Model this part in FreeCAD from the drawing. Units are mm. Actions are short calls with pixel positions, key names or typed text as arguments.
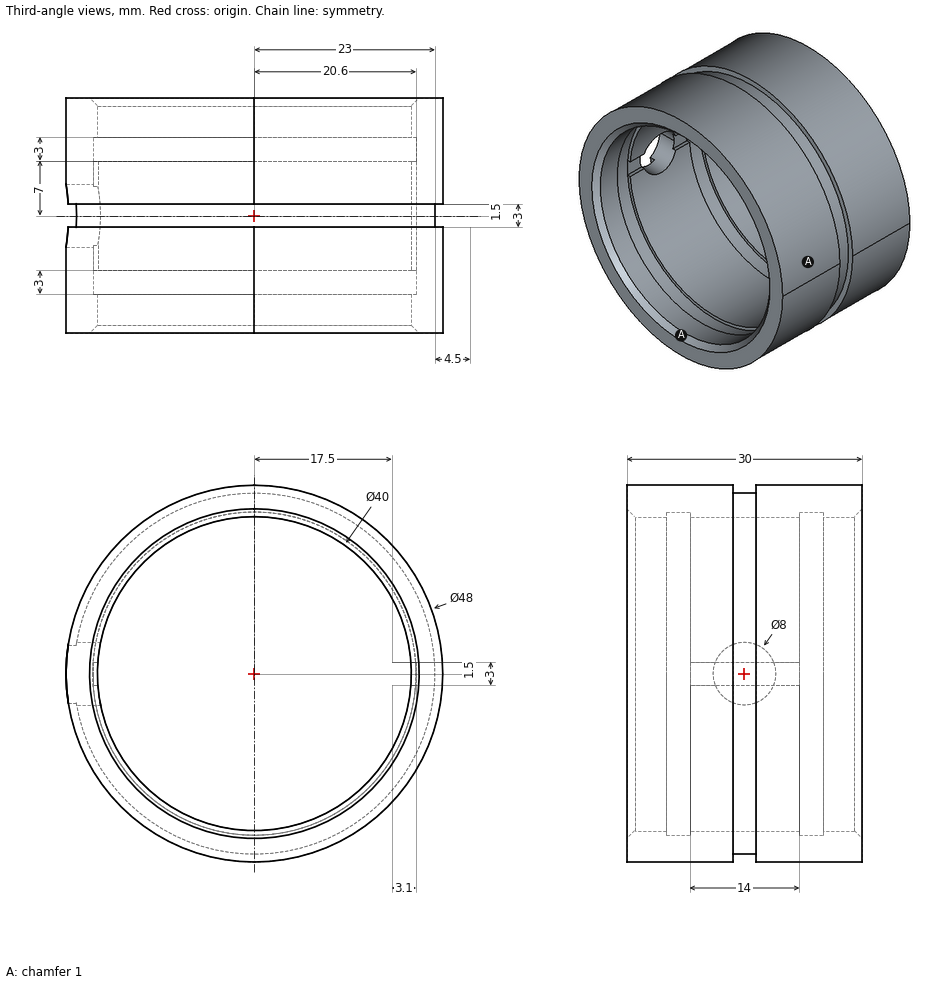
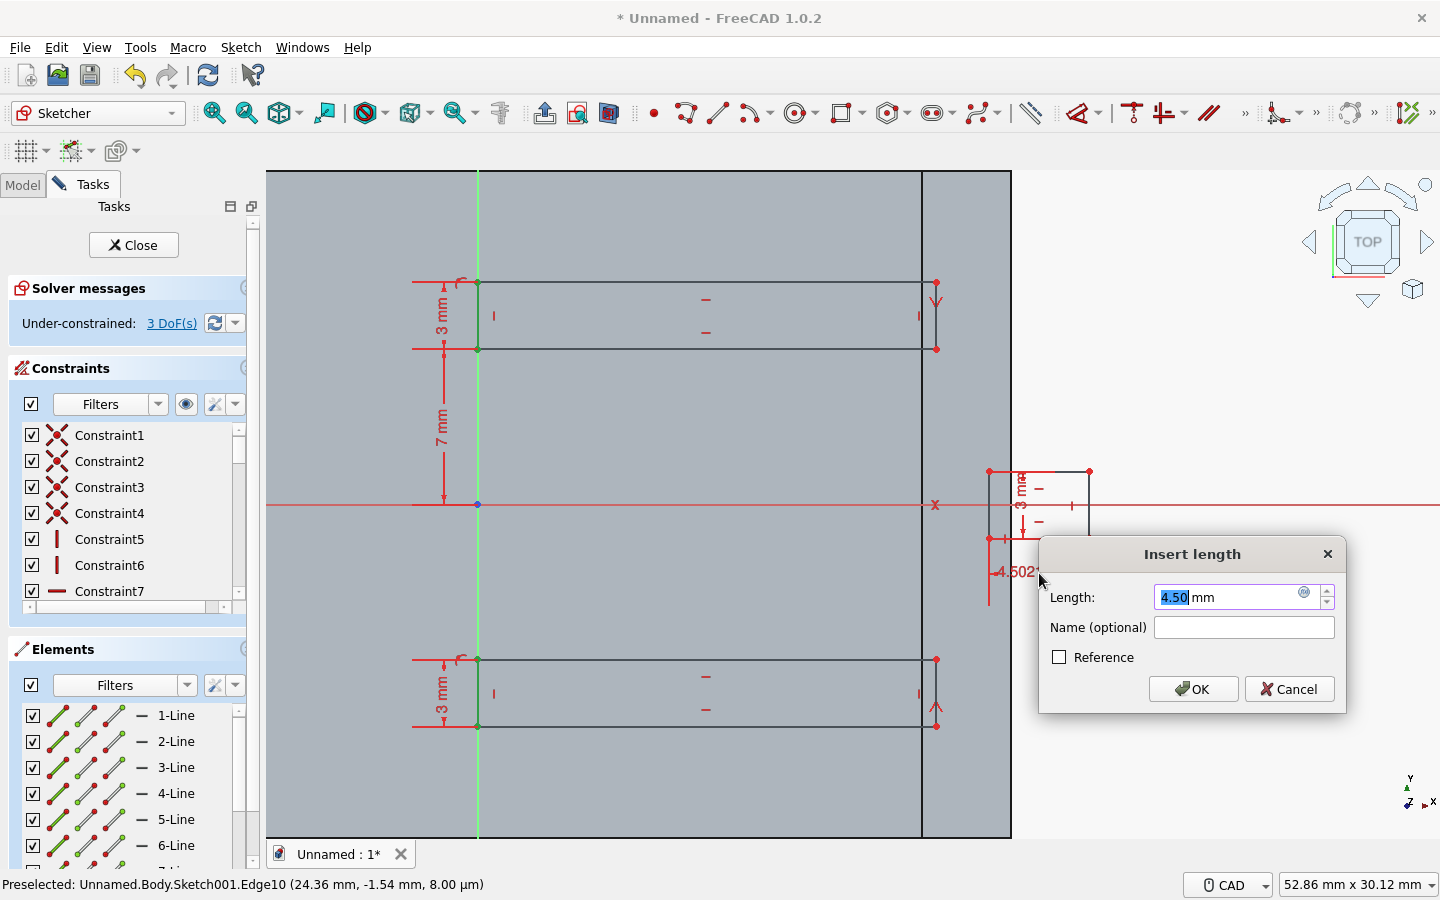
text(4.5)
key(Return)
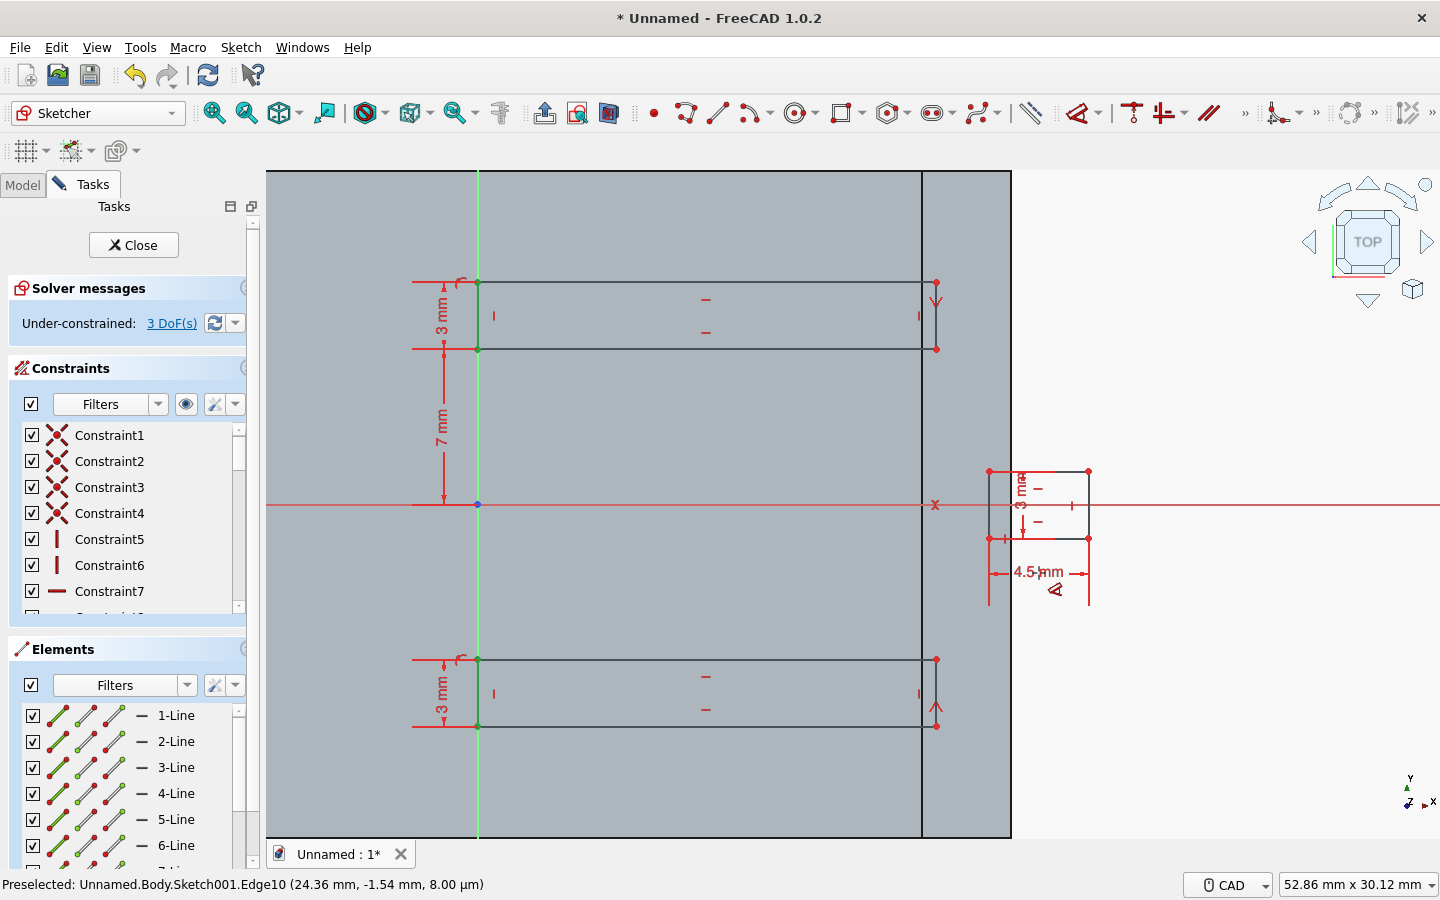
click(989, 472)
click(733, 438)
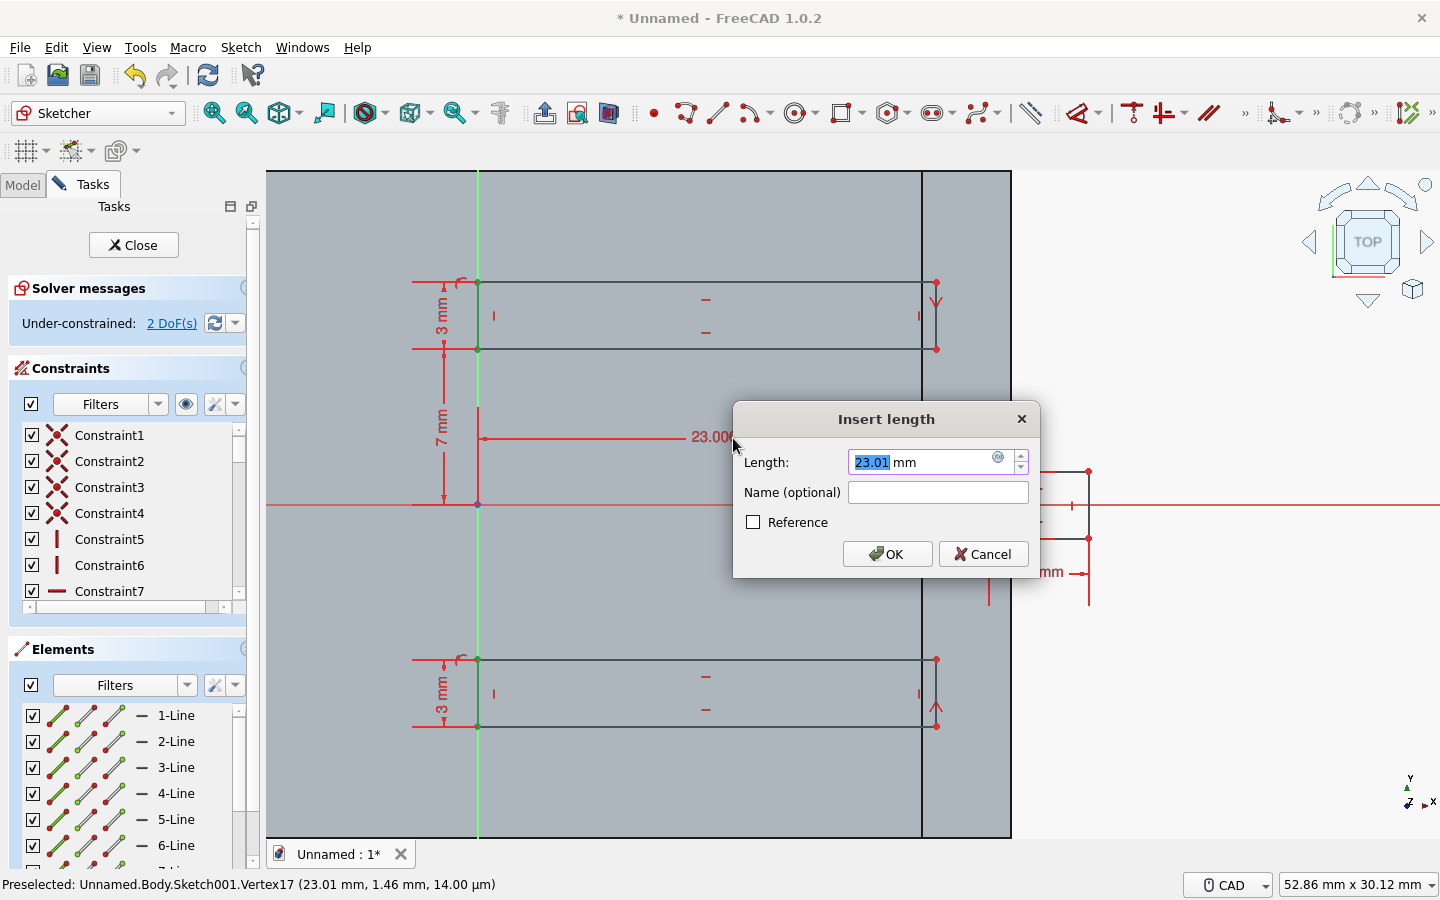
text(23)
key(Return)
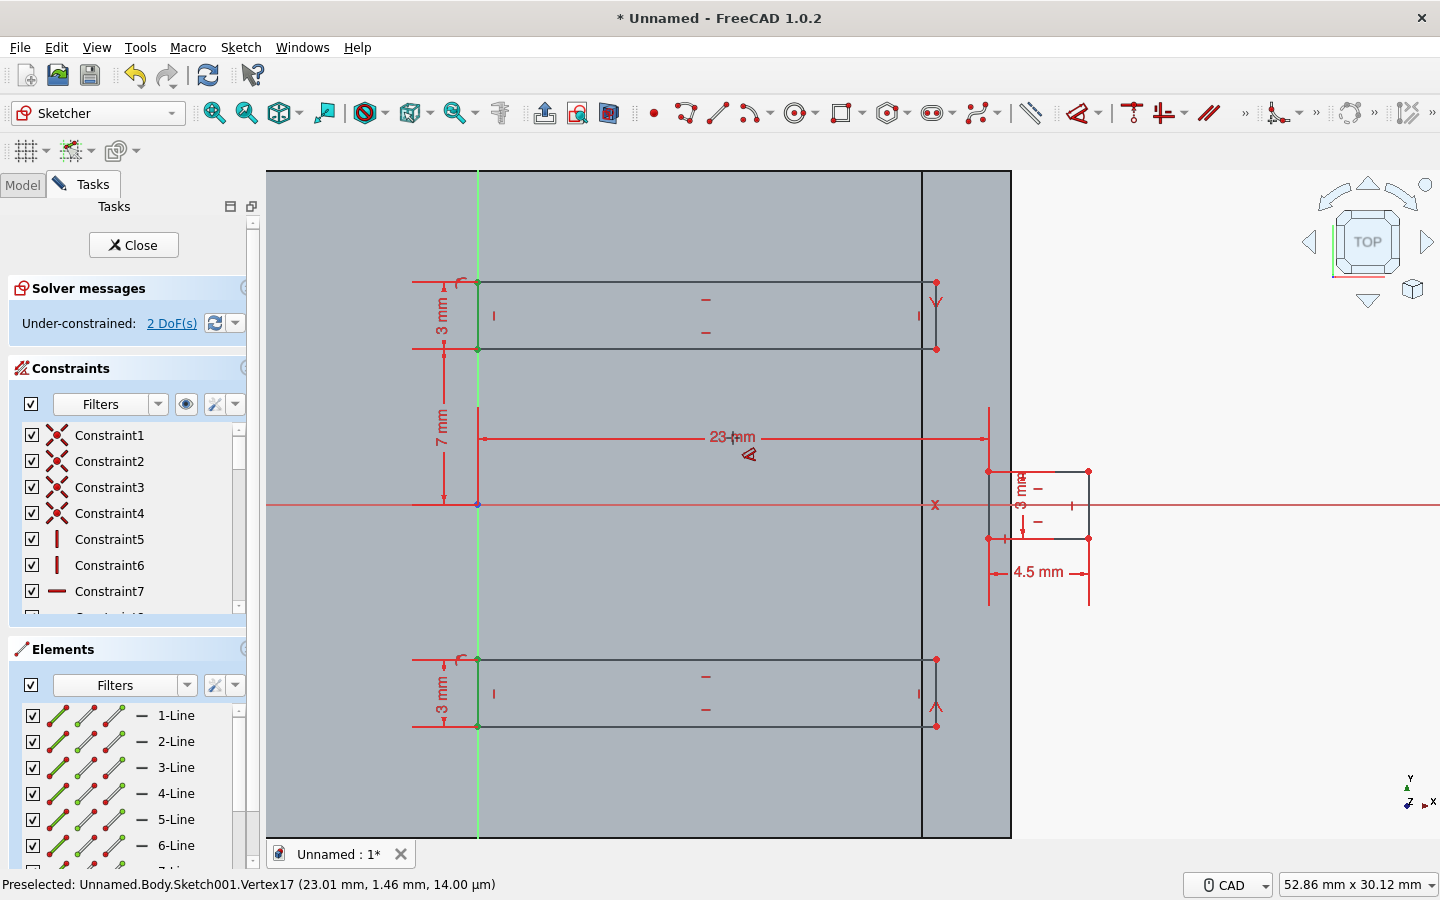
click(615, 349)
click(707, 315)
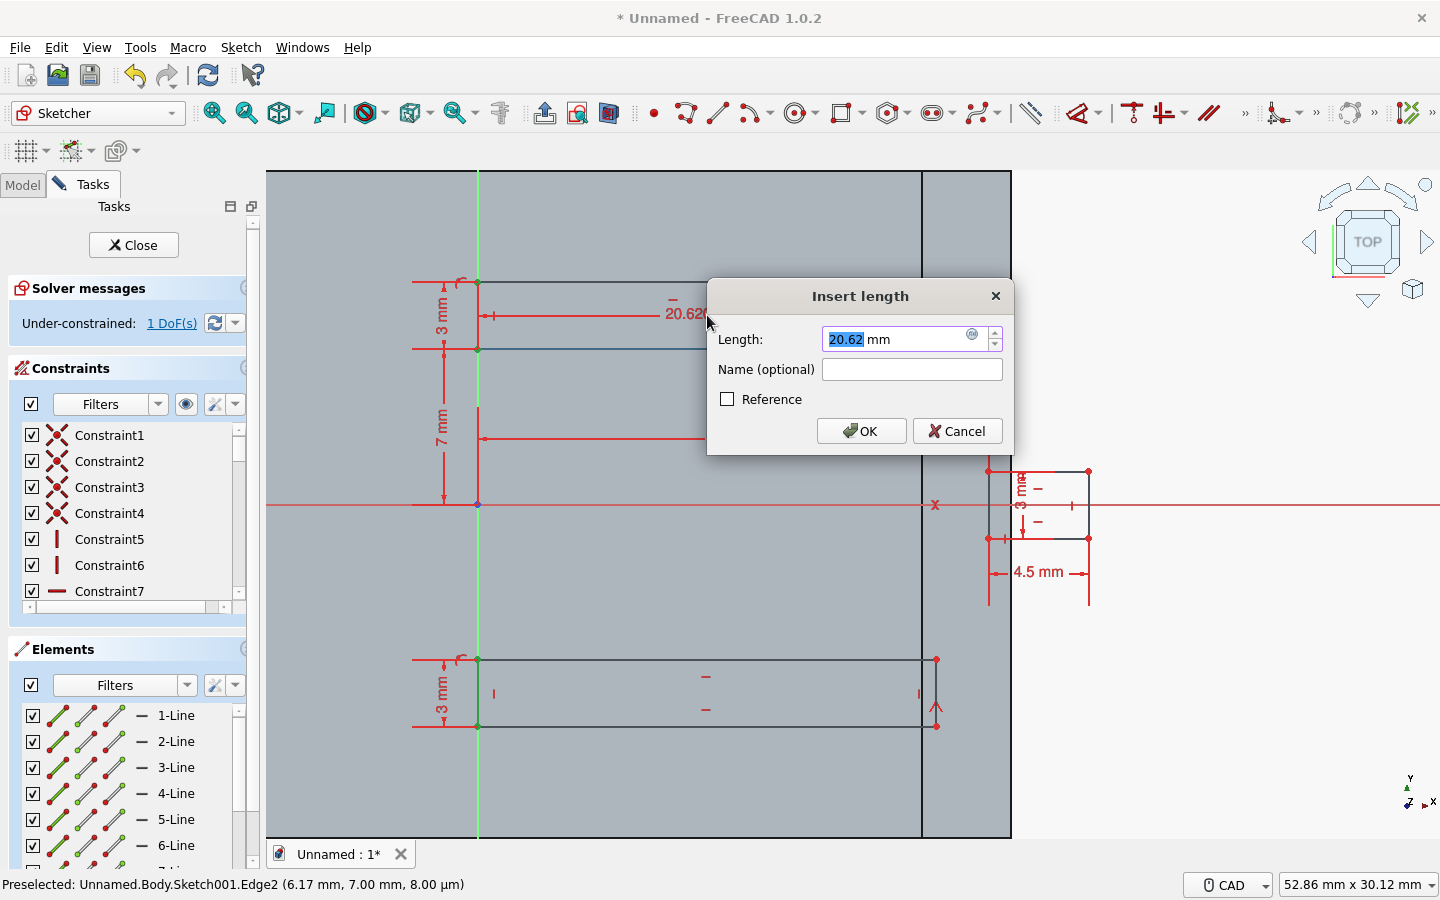
text(20.6)
key(Return)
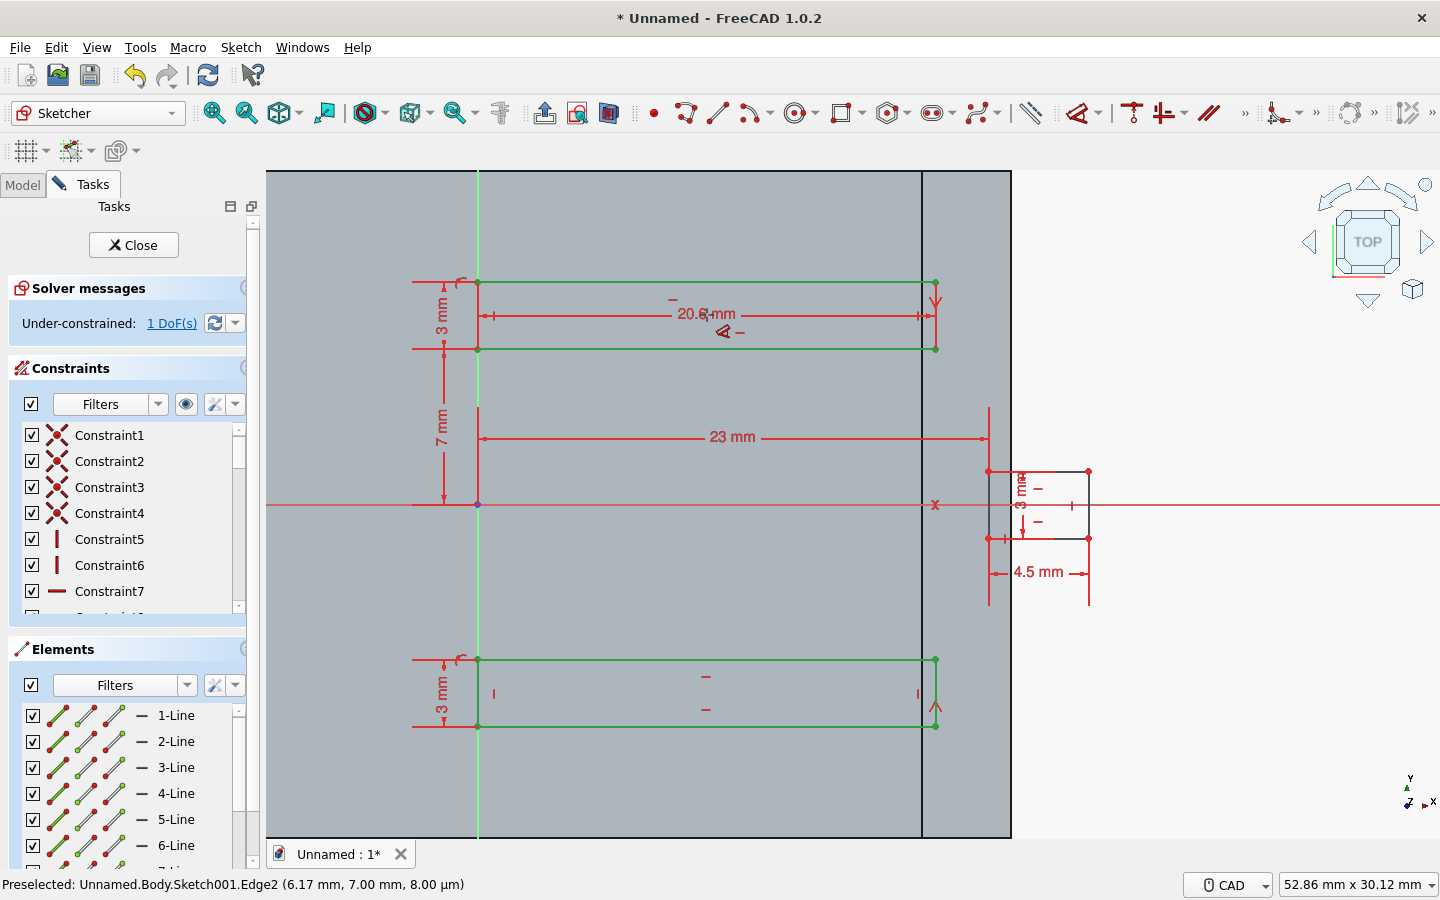
click(989, 472)
click(444, 488)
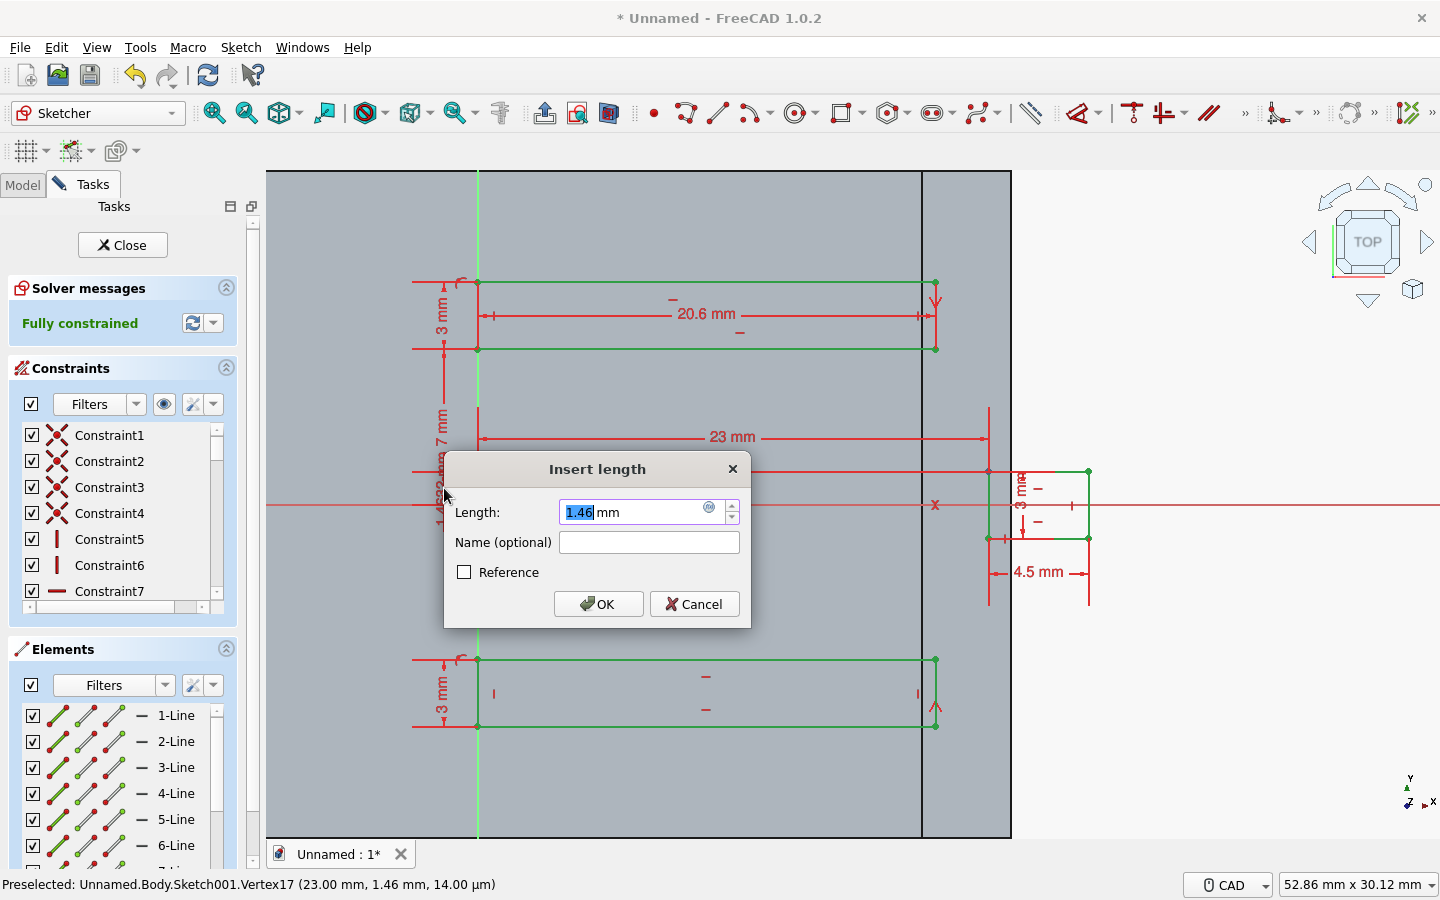
text(1.5)
key(Return)
key(Escape)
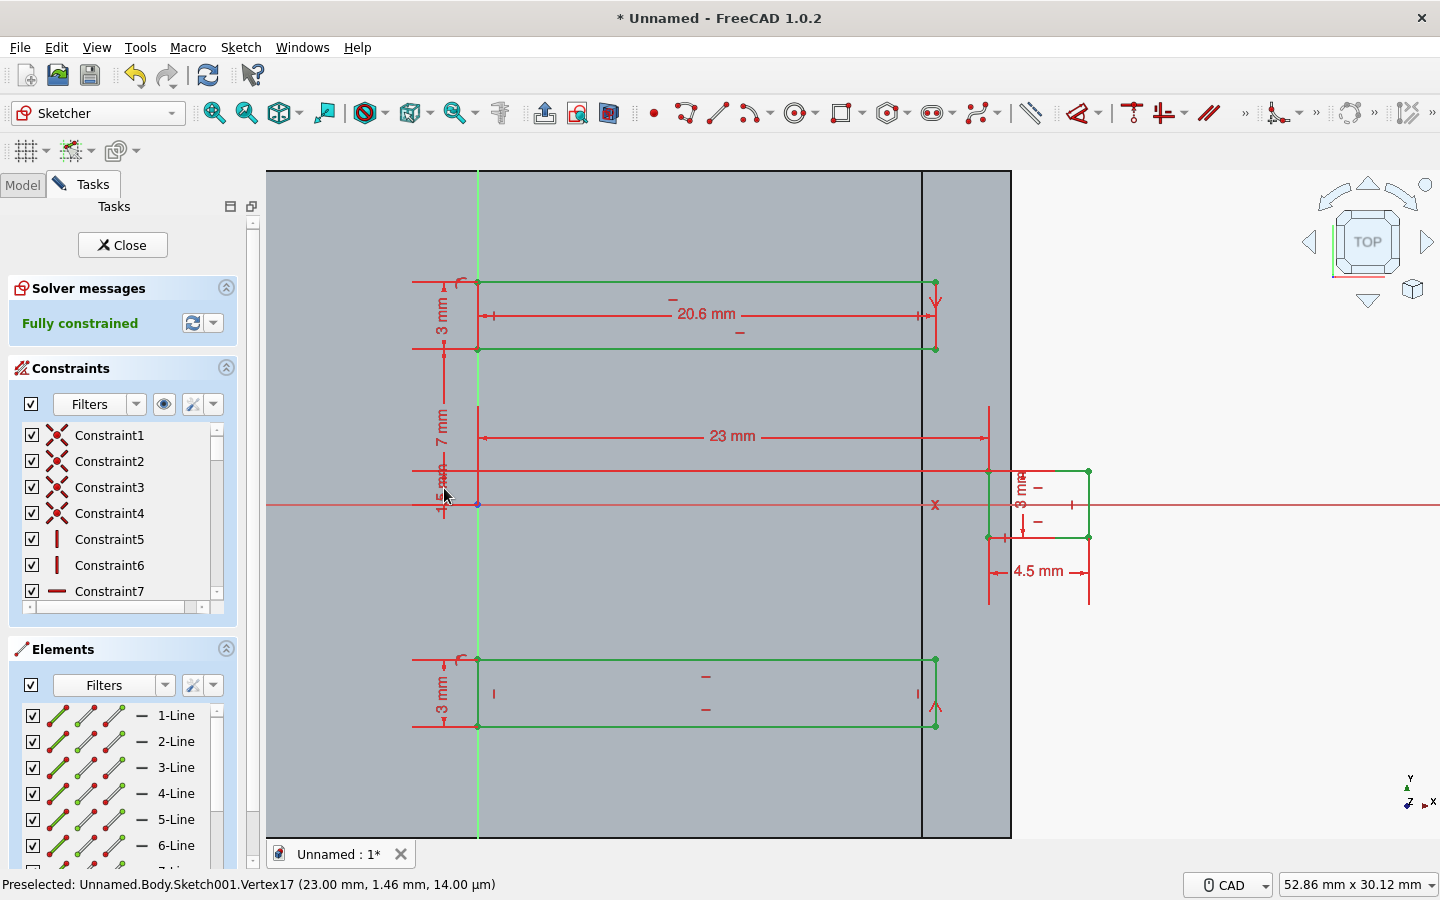
click(123, 245)